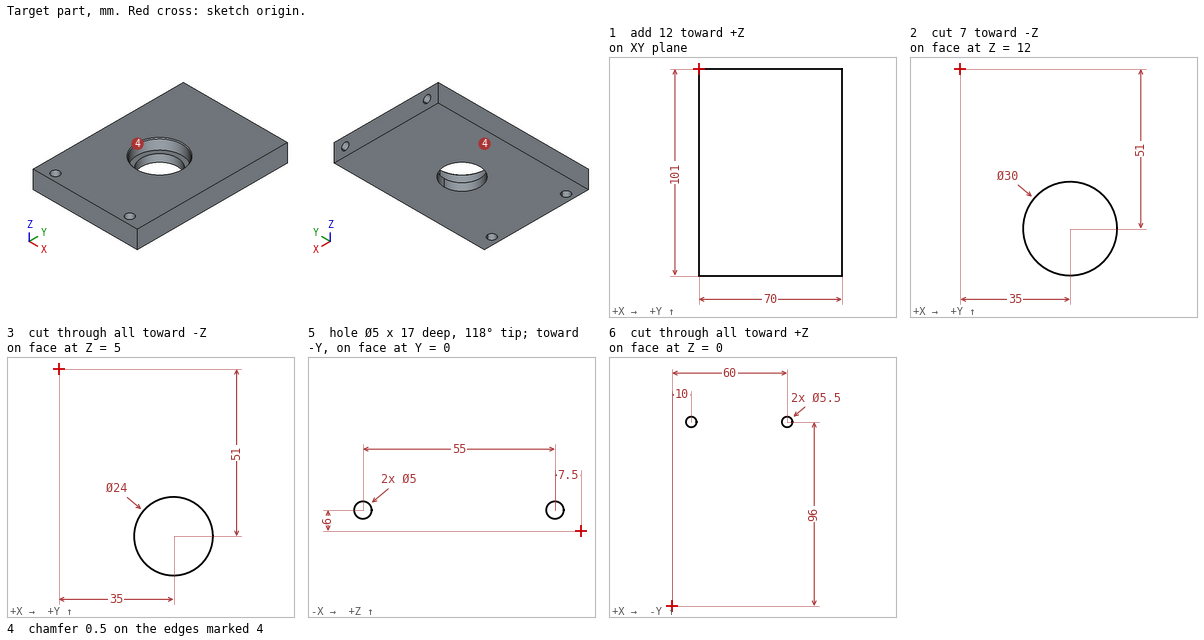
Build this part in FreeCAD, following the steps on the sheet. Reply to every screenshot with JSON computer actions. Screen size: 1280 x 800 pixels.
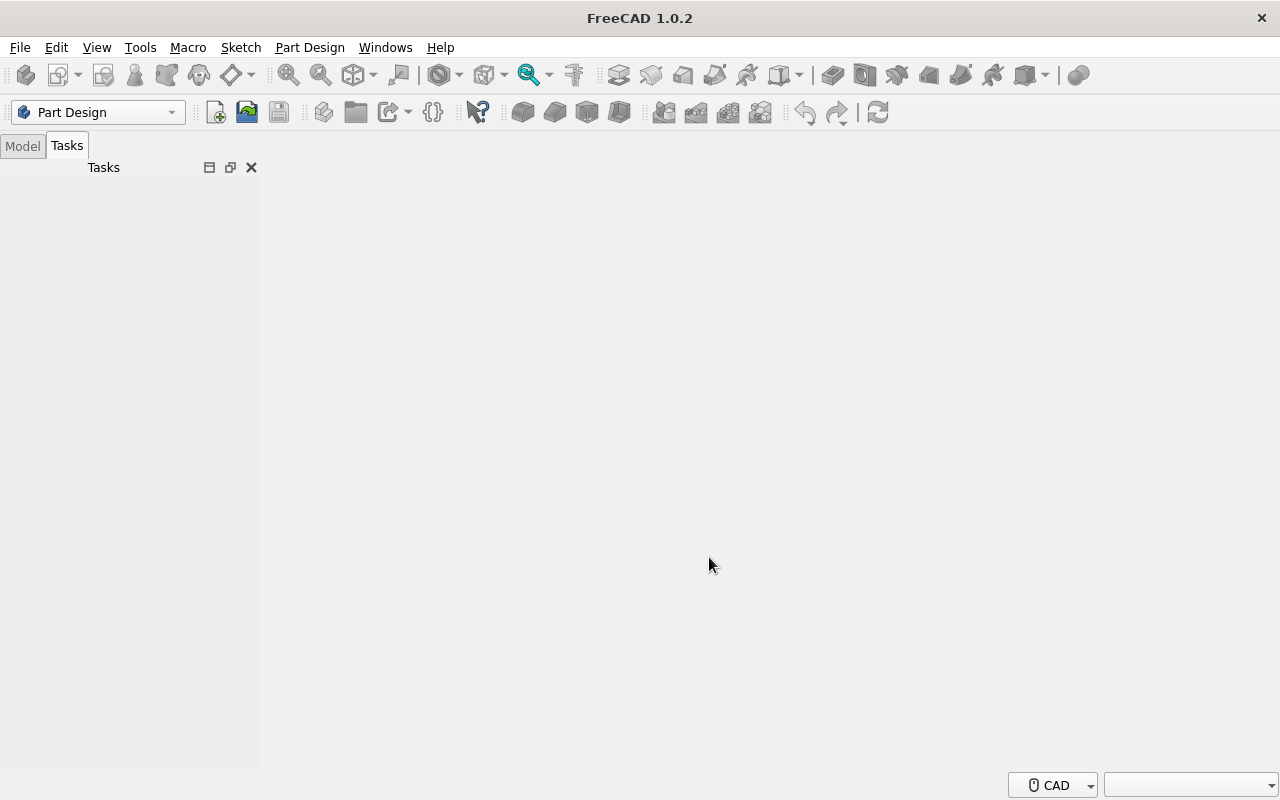
{"action": "left_click", "coordinate": [216, 112]}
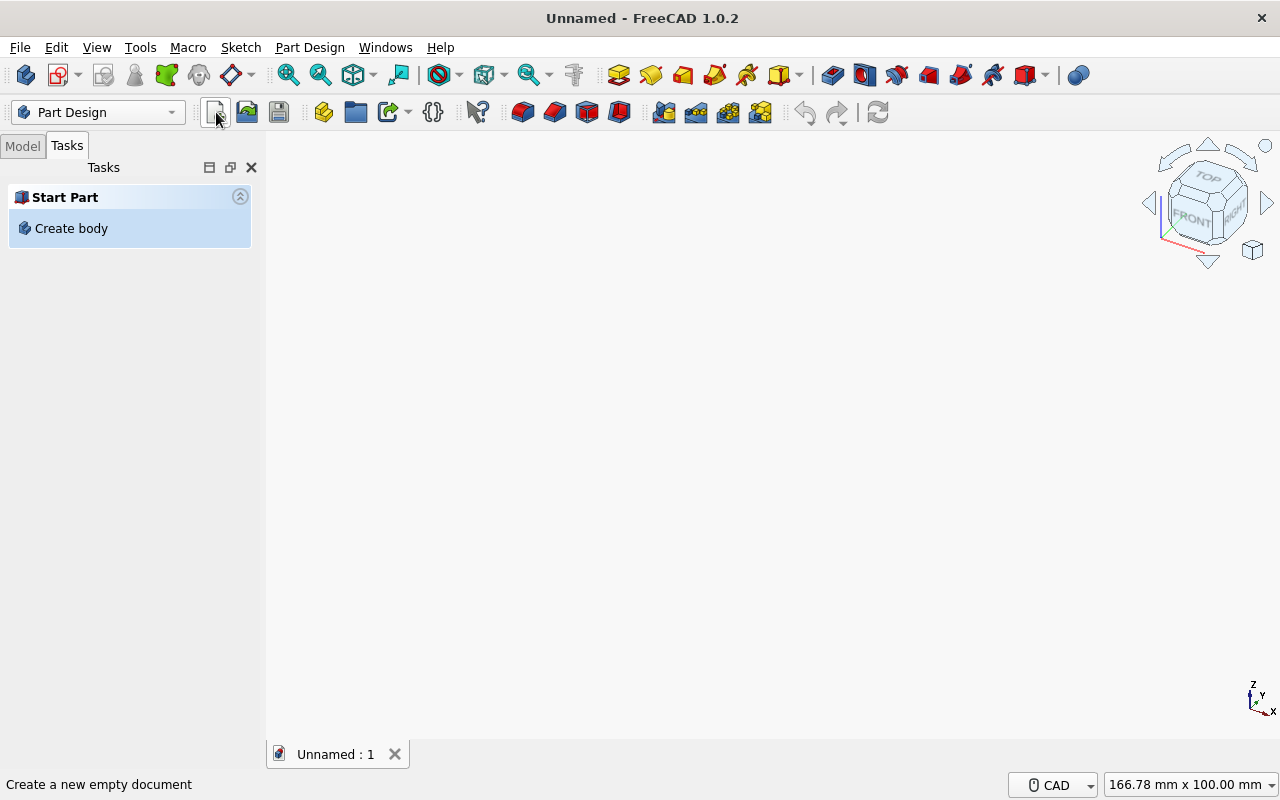
{"action": "left_click", "coordinate": [58, 76]}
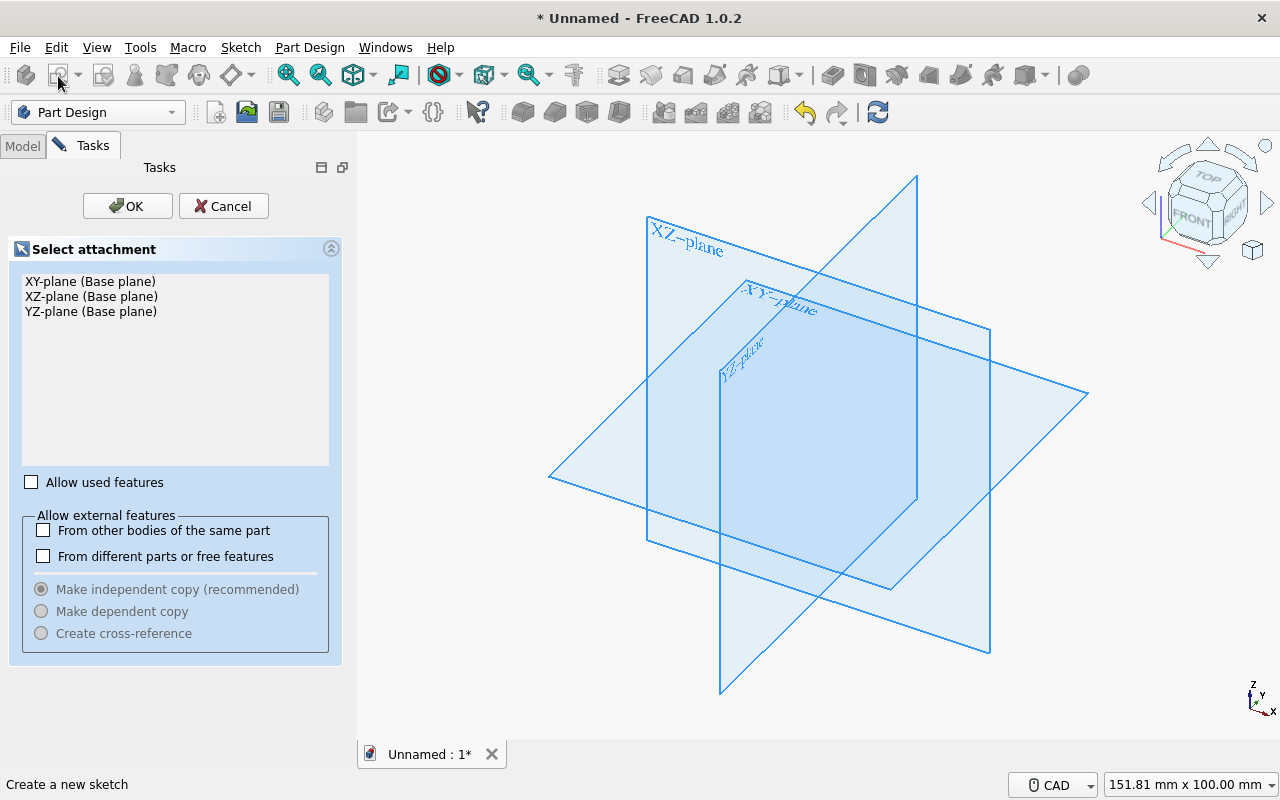
{"action": "left_click", "coordinate": [82, 282]}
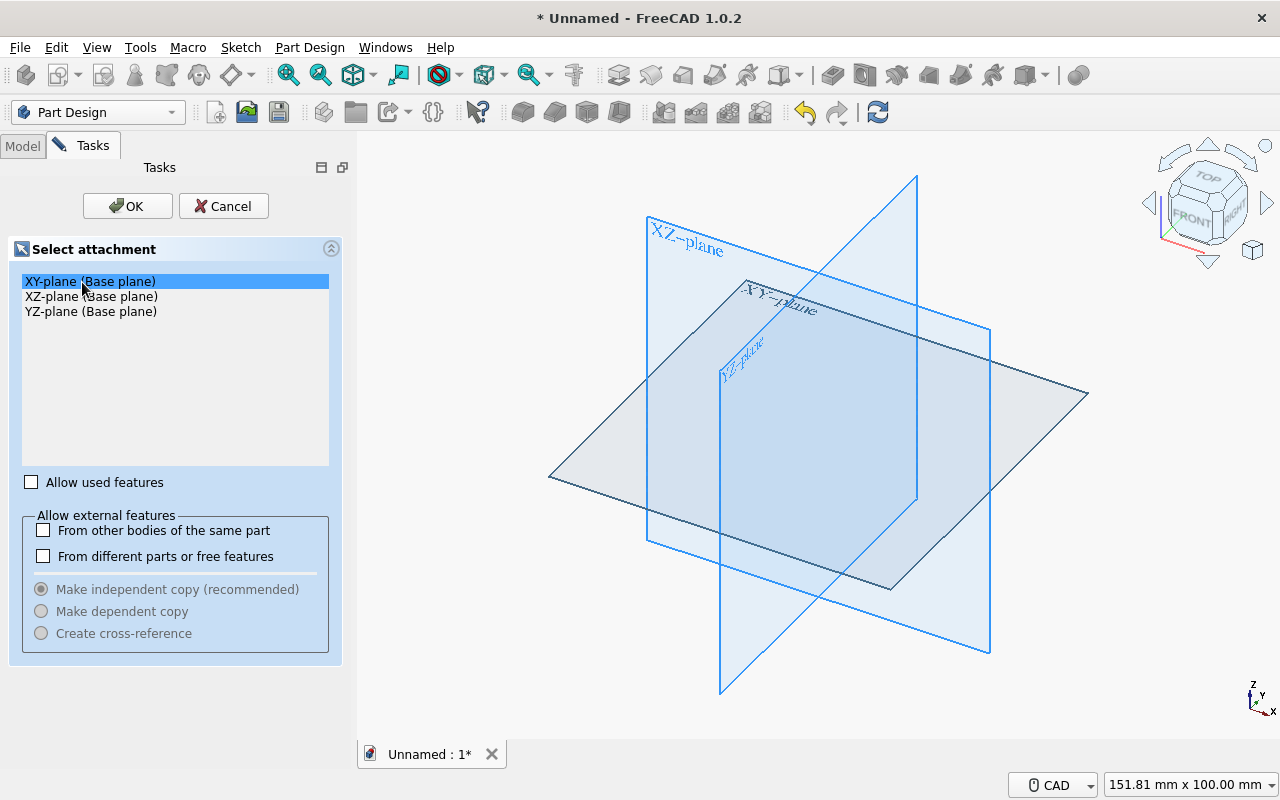
{"action": "left_click", "coordinate": [128, 206]}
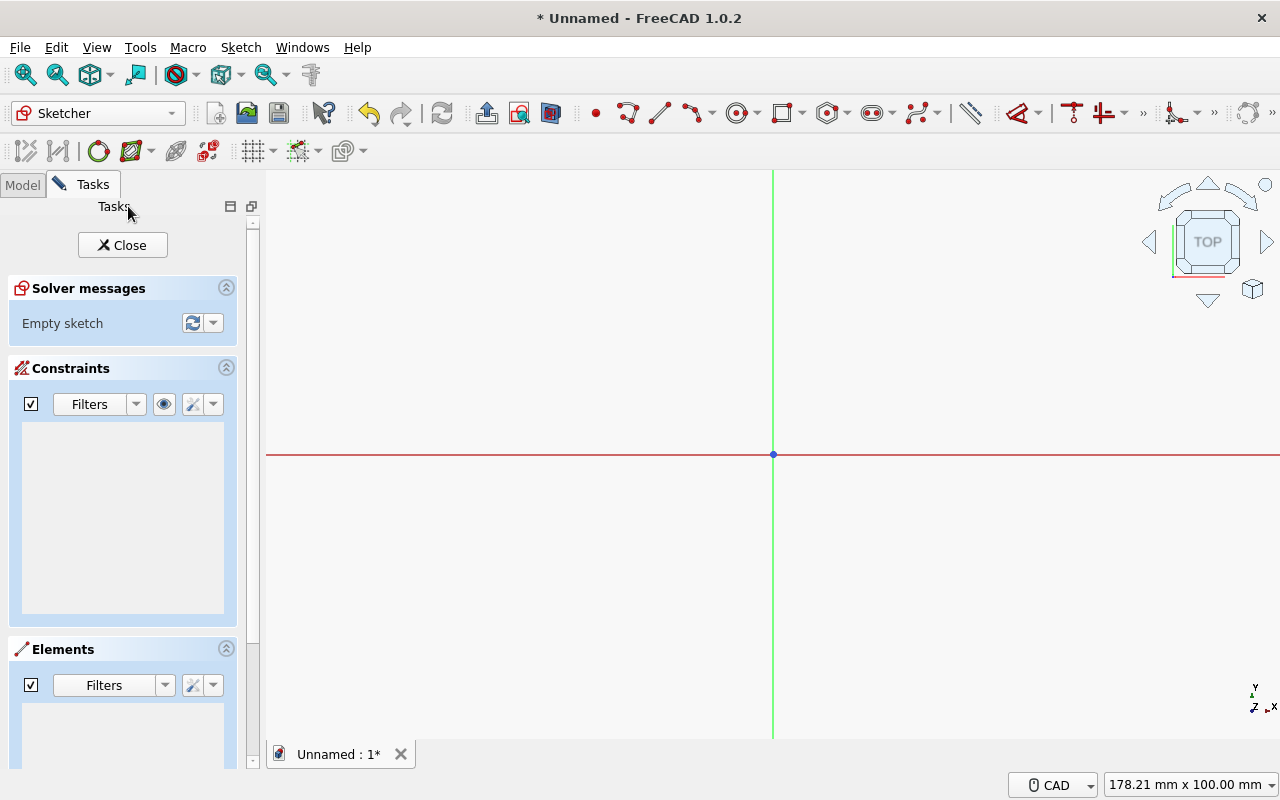
{"action": "scroll", "coordinate": [379, 198], "scroll_direction": "down", "scroll_amount": 3}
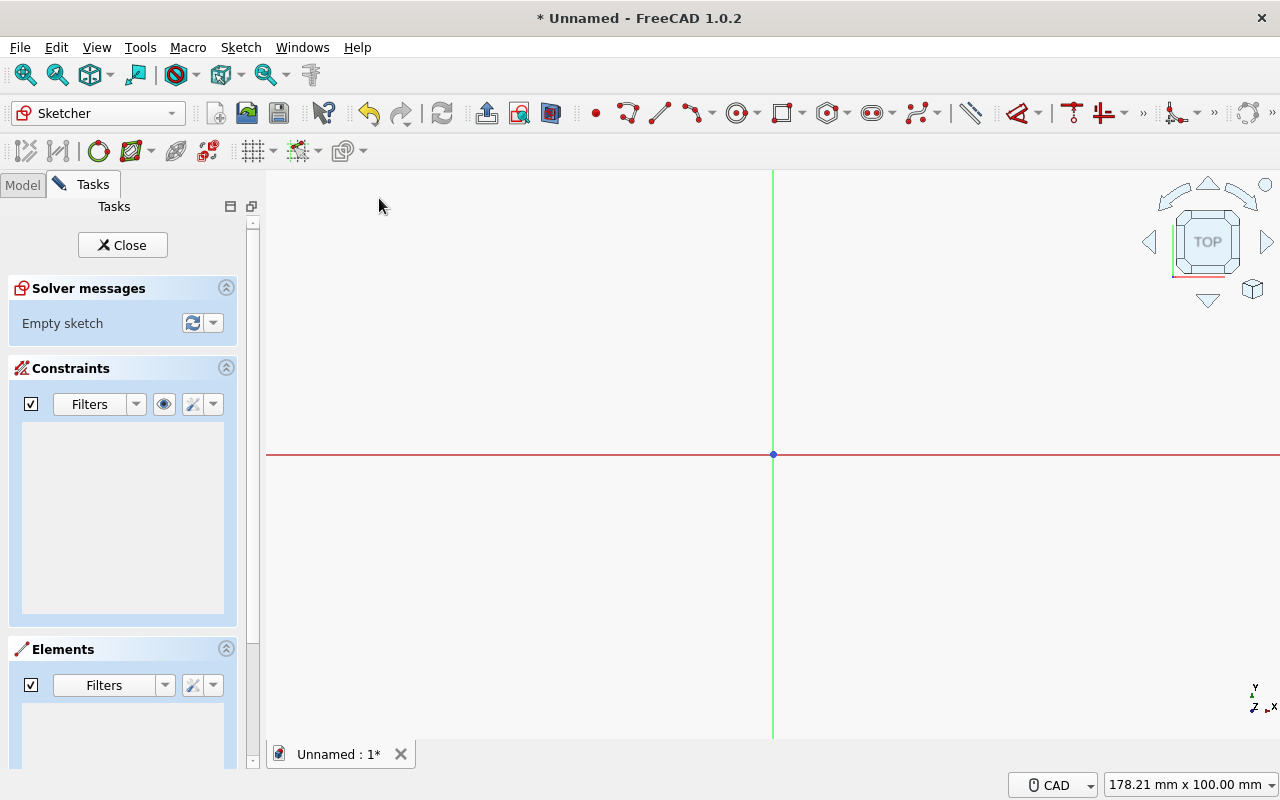
{"action": "left_click", "coordinate": [782, 114]}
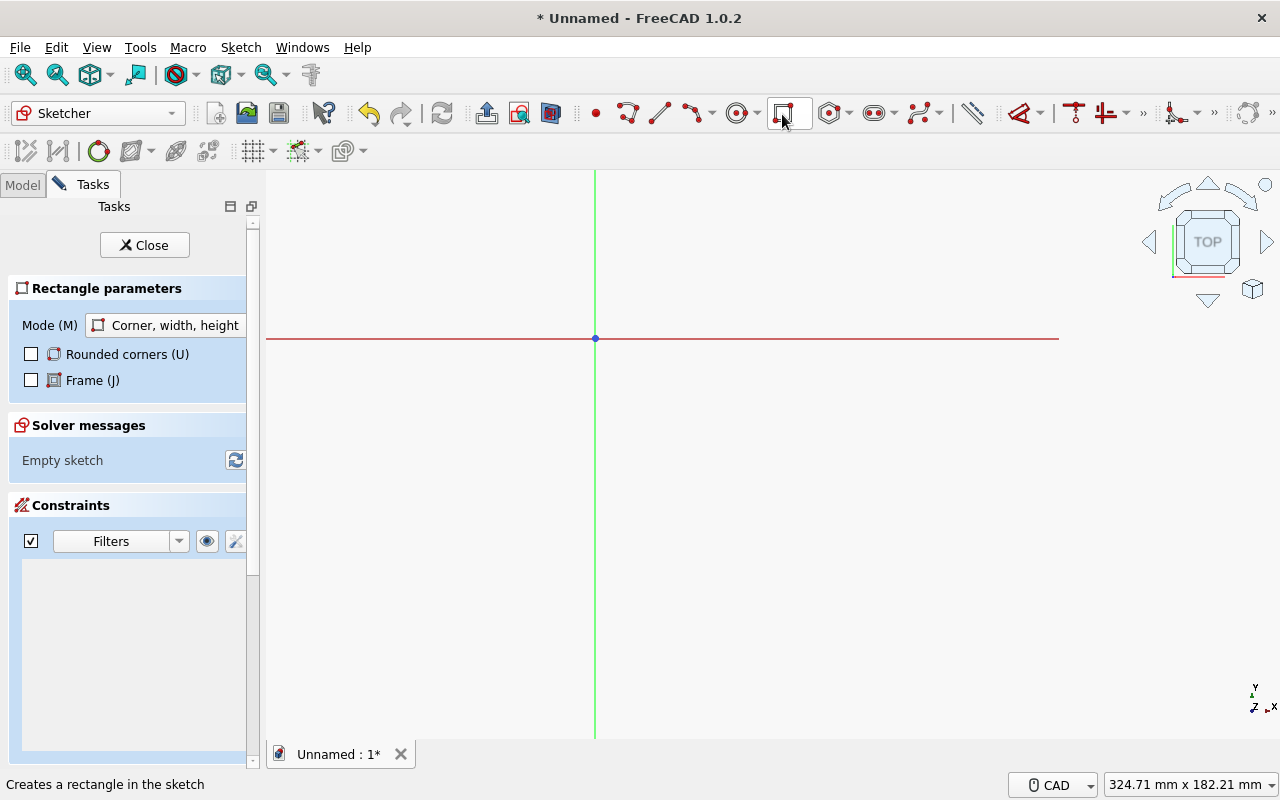
{"action": "left_click", "coordinate": [595, 339]}
{"action": "left_click", "coordinate": [814, 654]}
{"action": "key", "text": "Escape"}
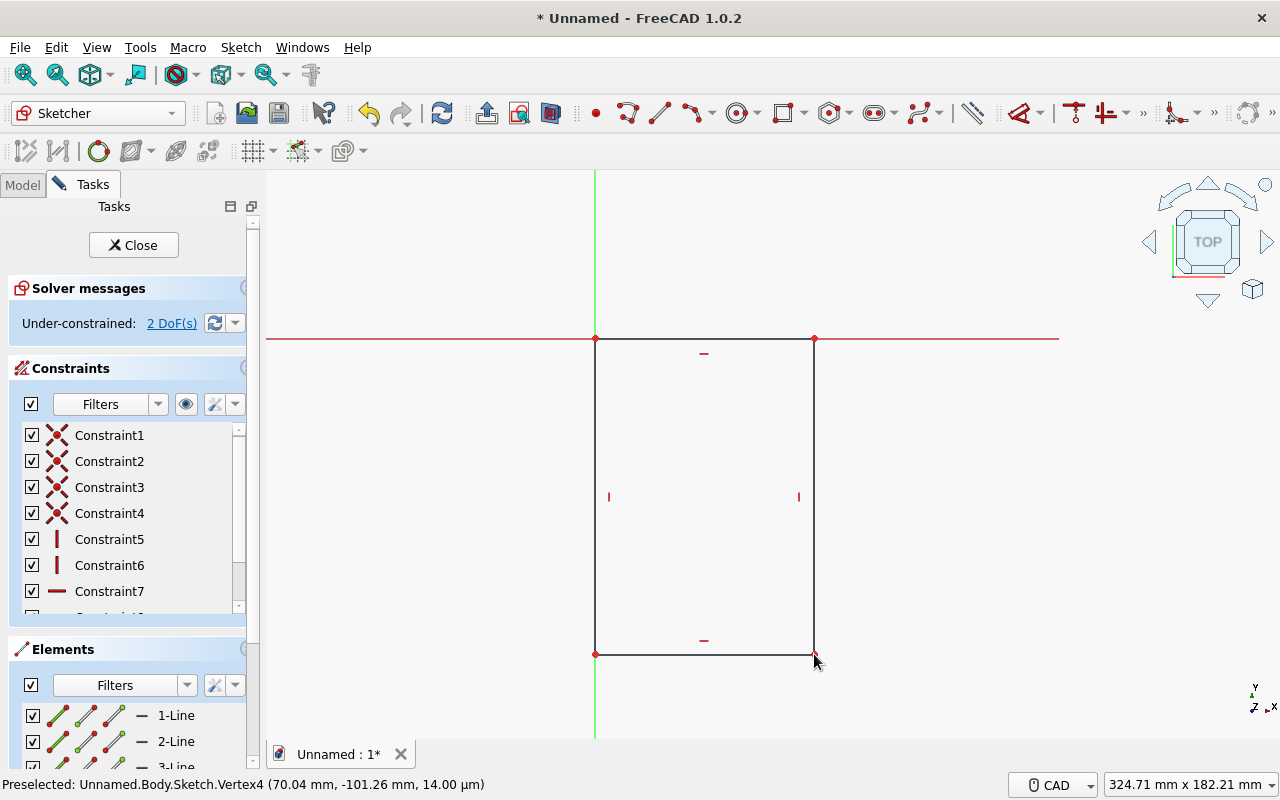
{"action": "left_click", "coordinate": [661, 655]}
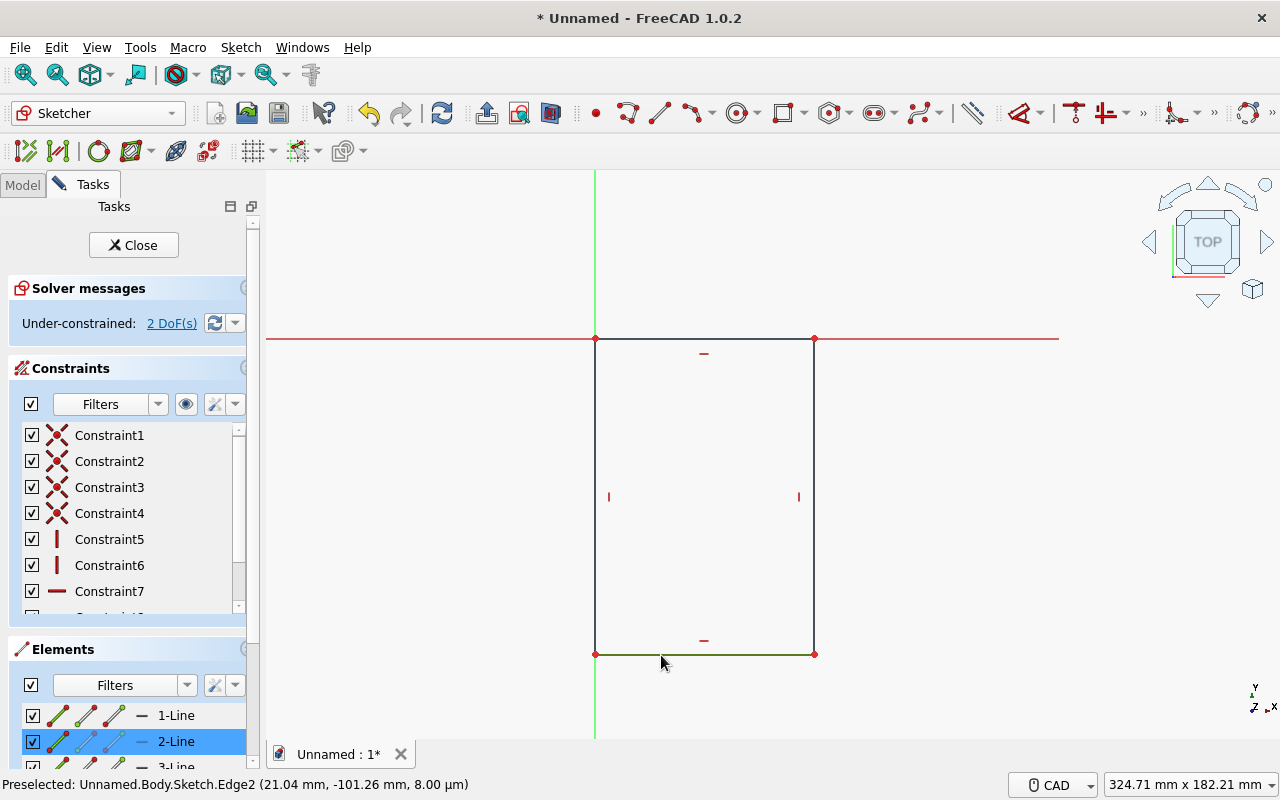
{"action": "left_click", "coordinate": [1042, 114]}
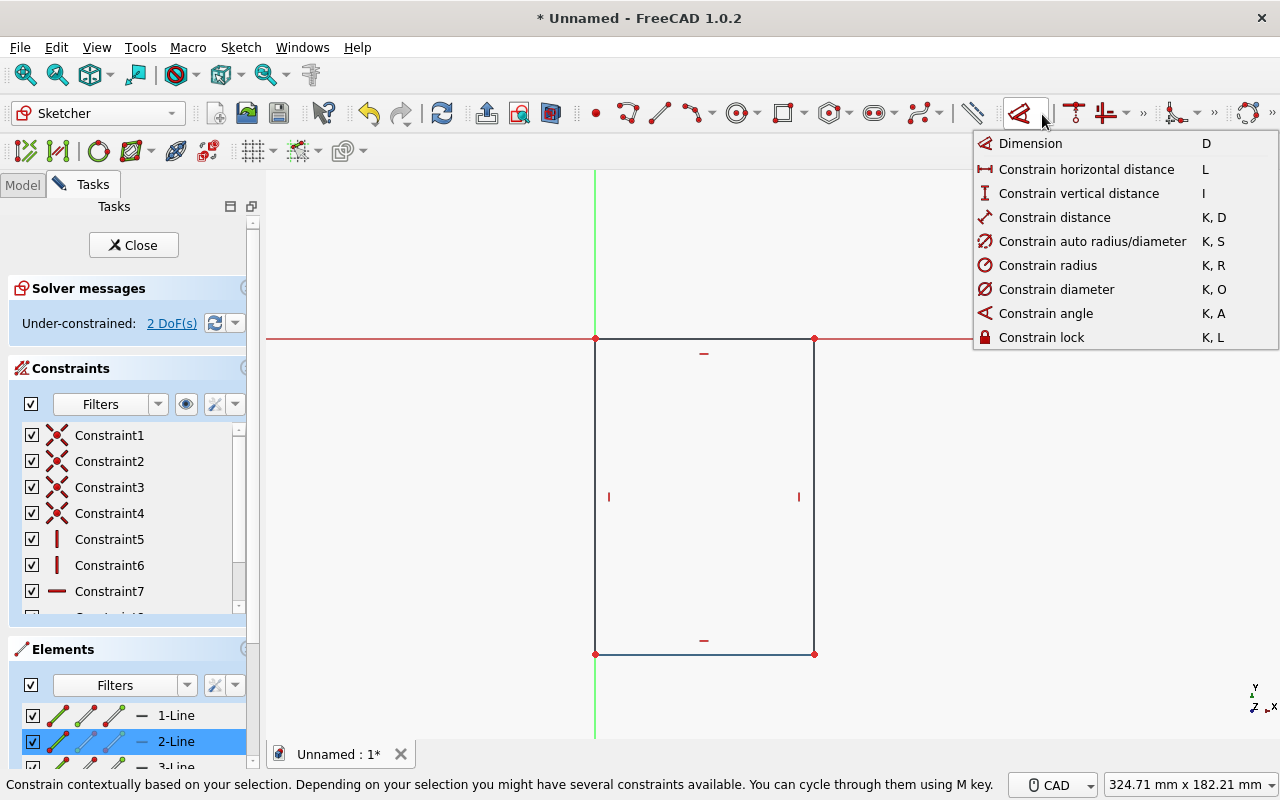
{"action": "left_click", "coordinate": [1126, 169]}